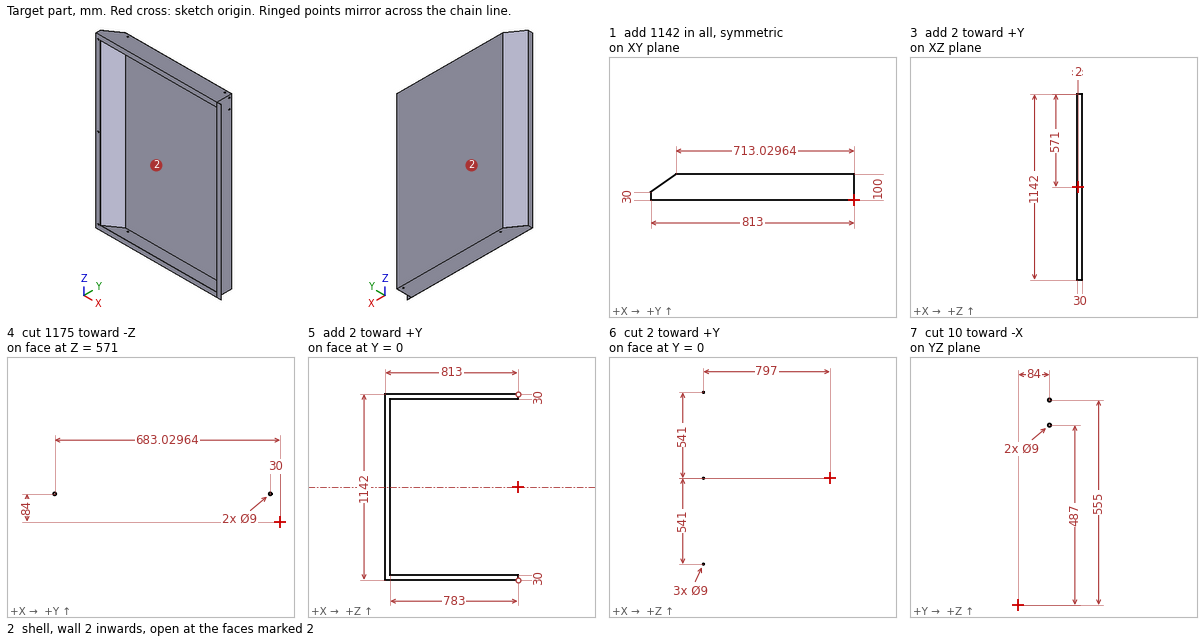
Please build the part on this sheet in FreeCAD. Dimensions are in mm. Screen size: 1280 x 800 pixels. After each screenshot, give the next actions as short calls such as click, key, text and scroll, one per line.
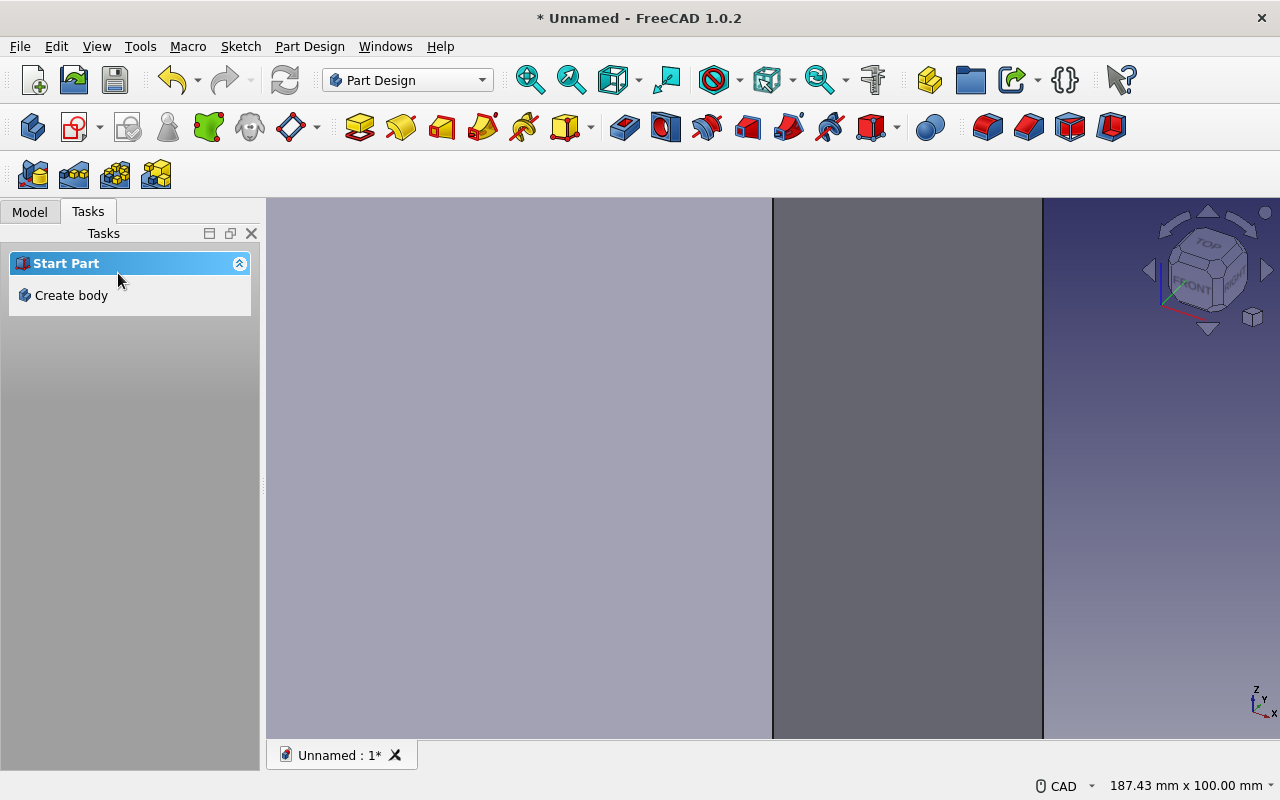
click(531, 80)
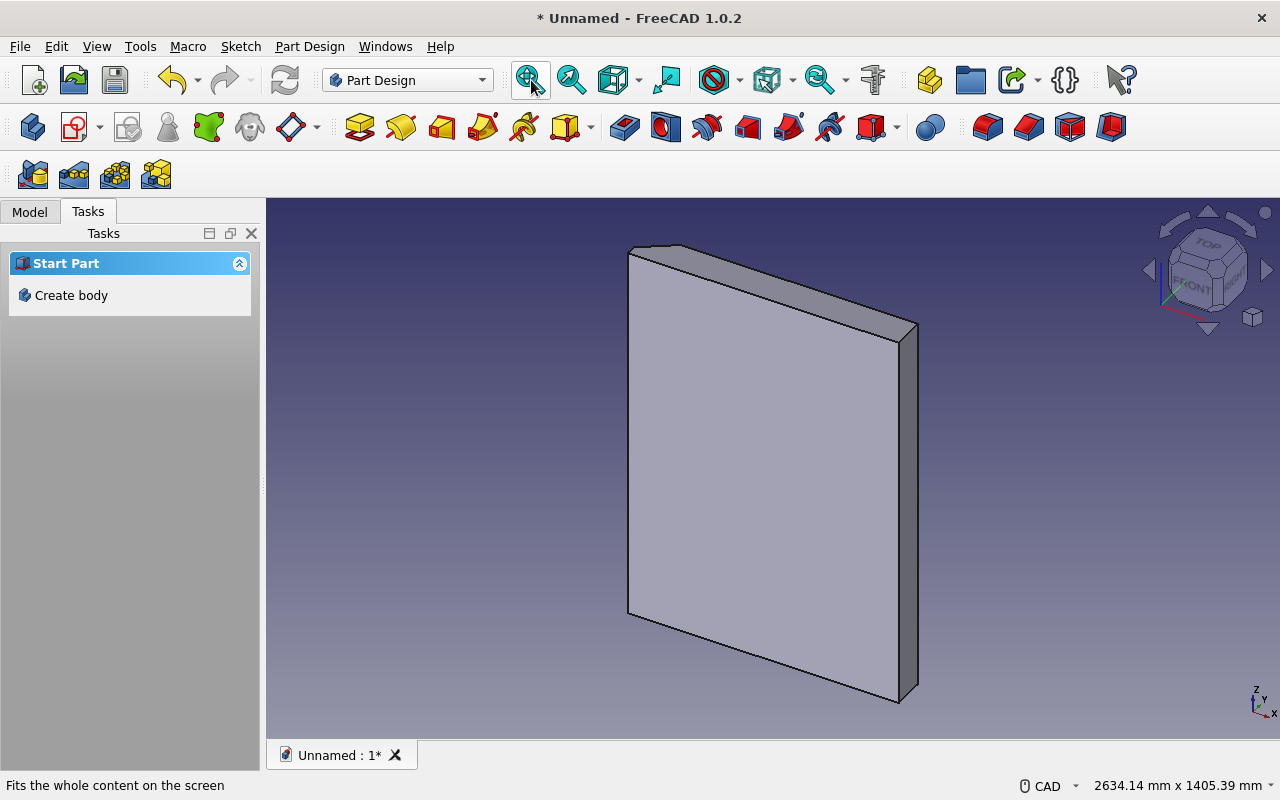
click(763, 426)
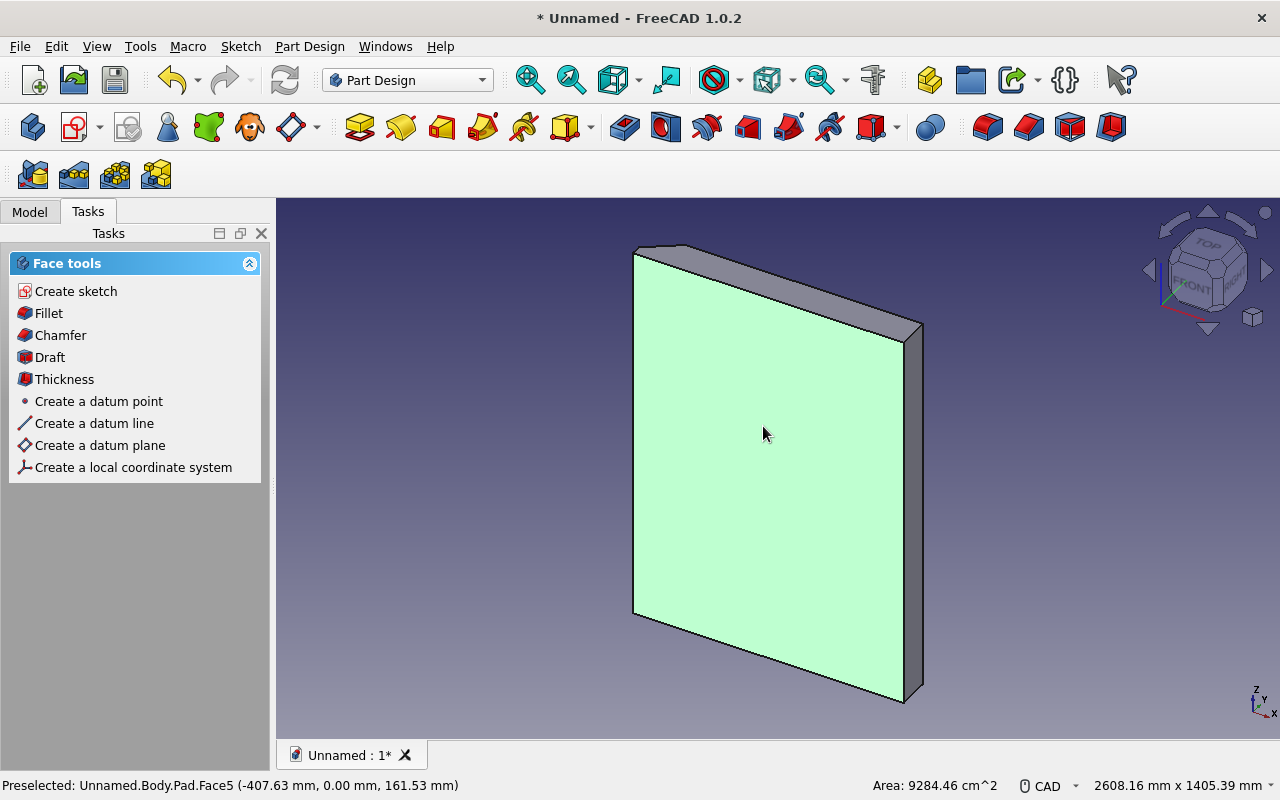
click(1111, 128)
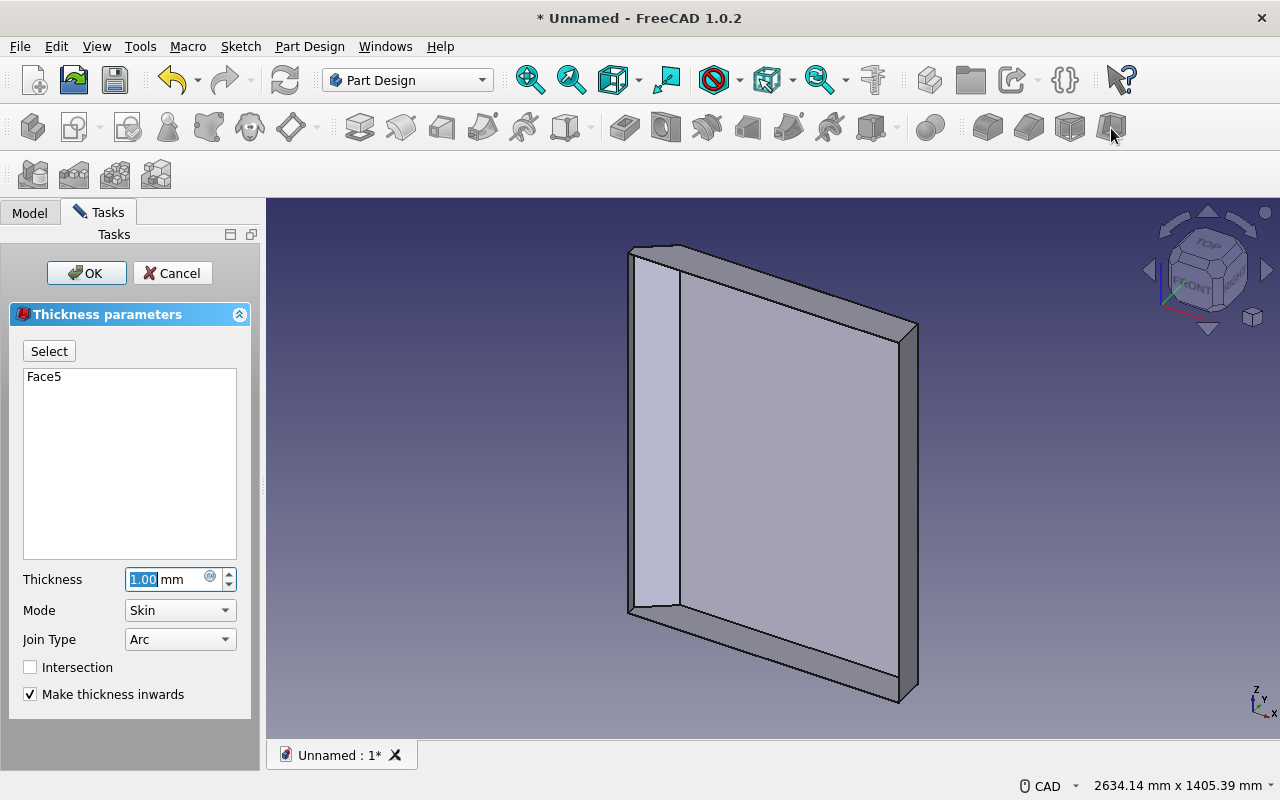
text(2)
key(Tab)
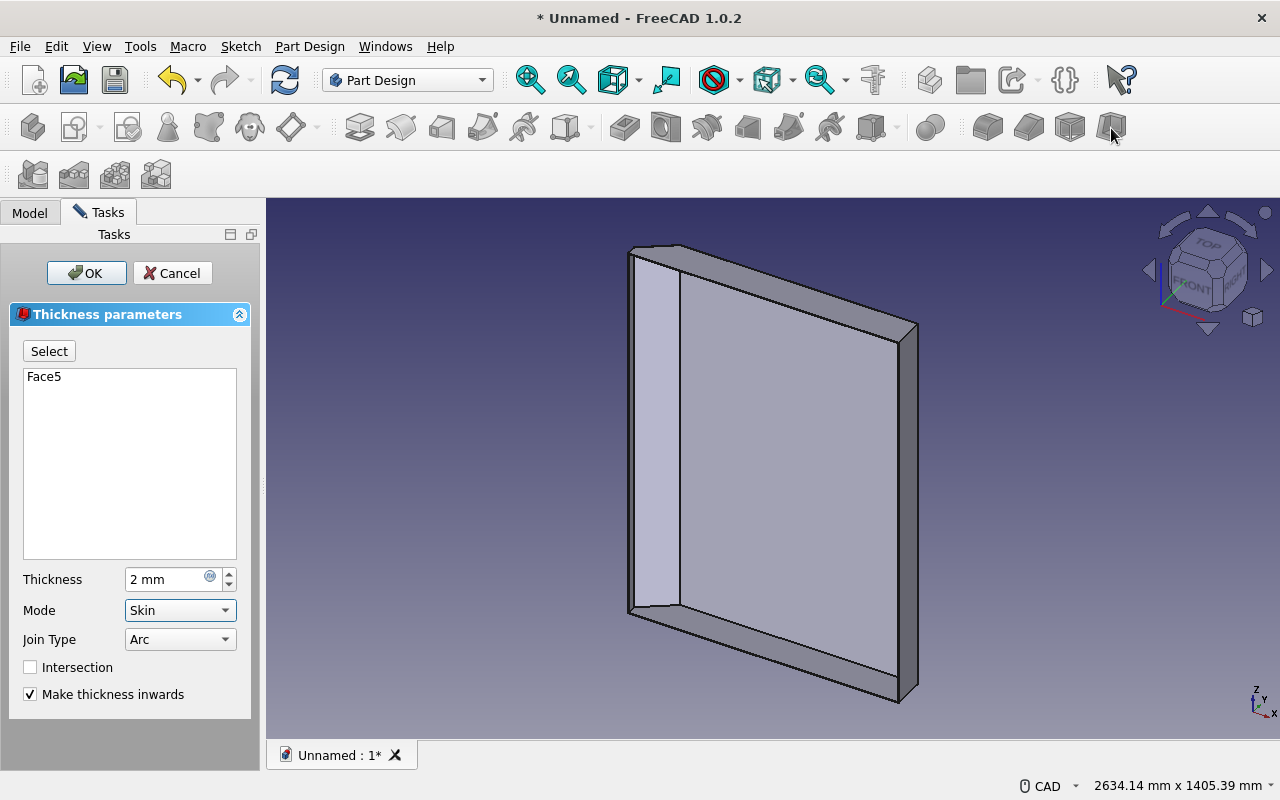
click(181, 640)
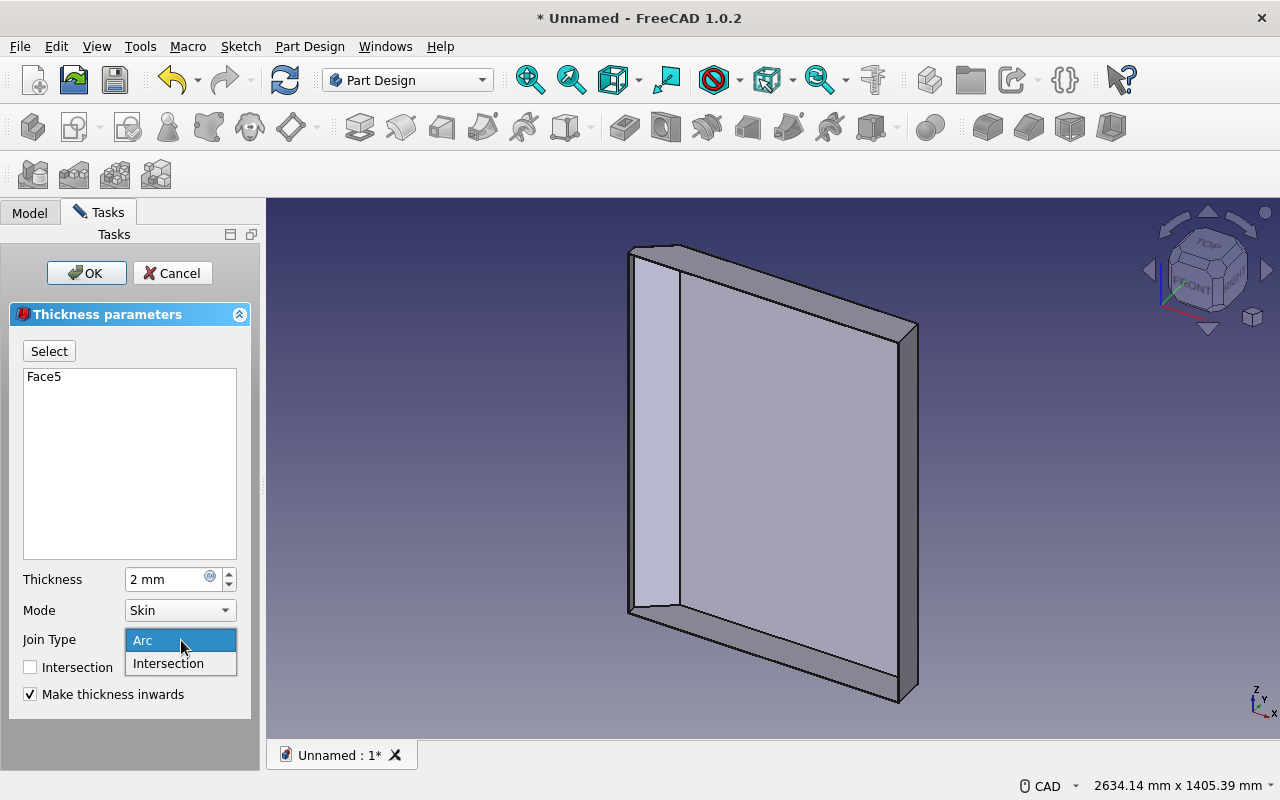
click(179, 664)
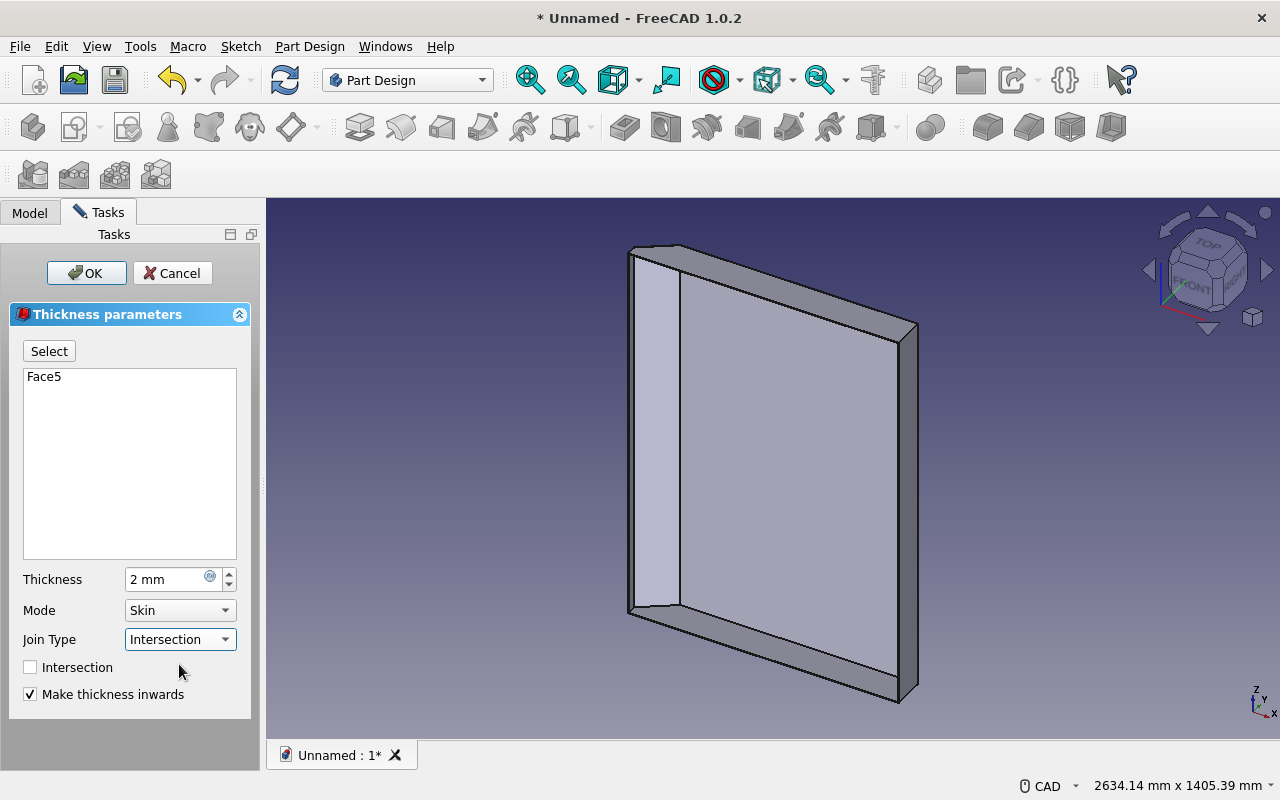
click(87, 273)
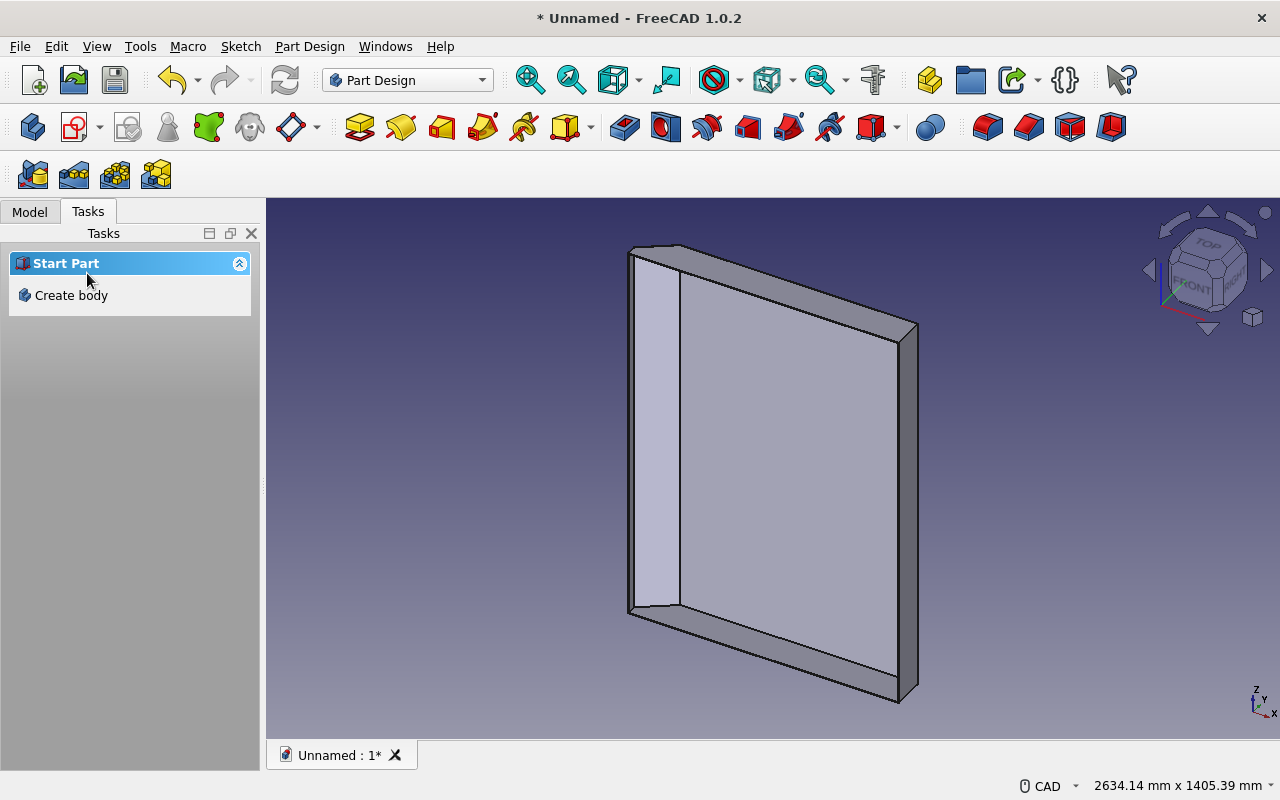
click(74, 128)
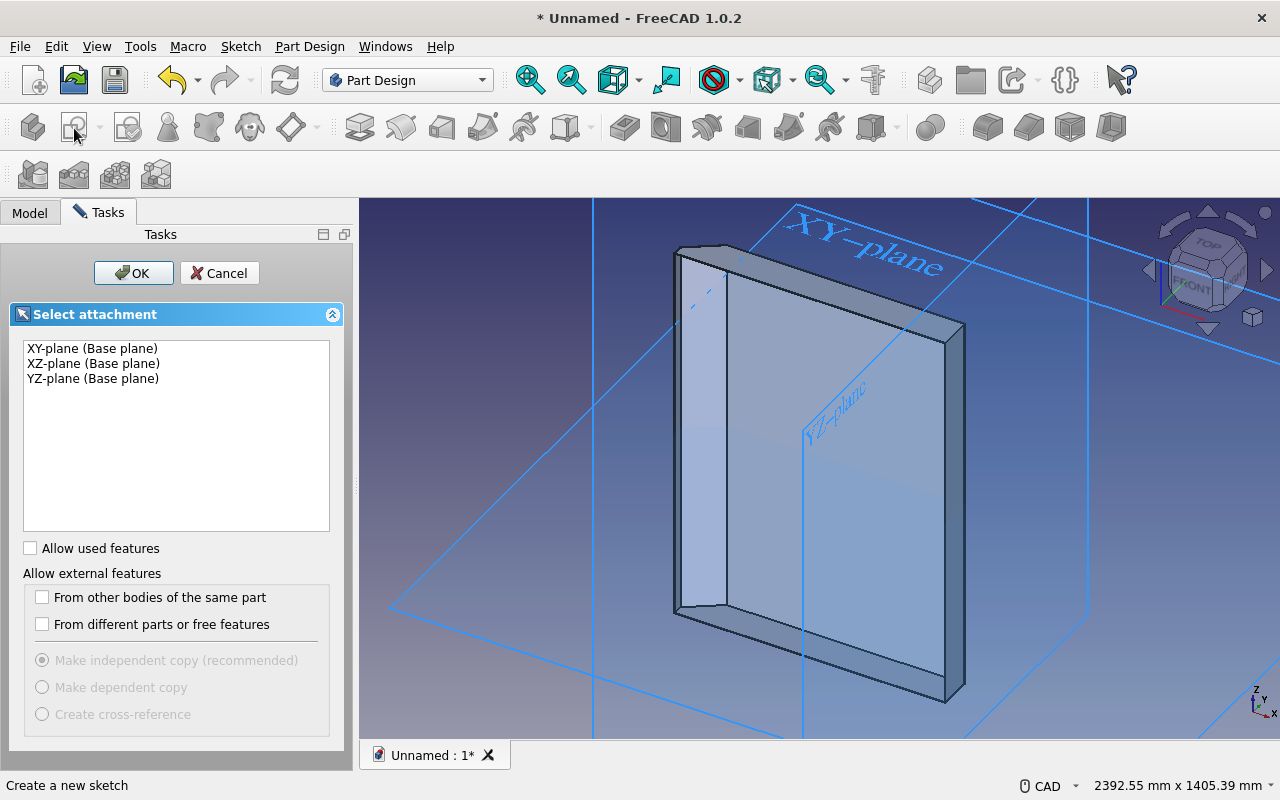
click(84, 364)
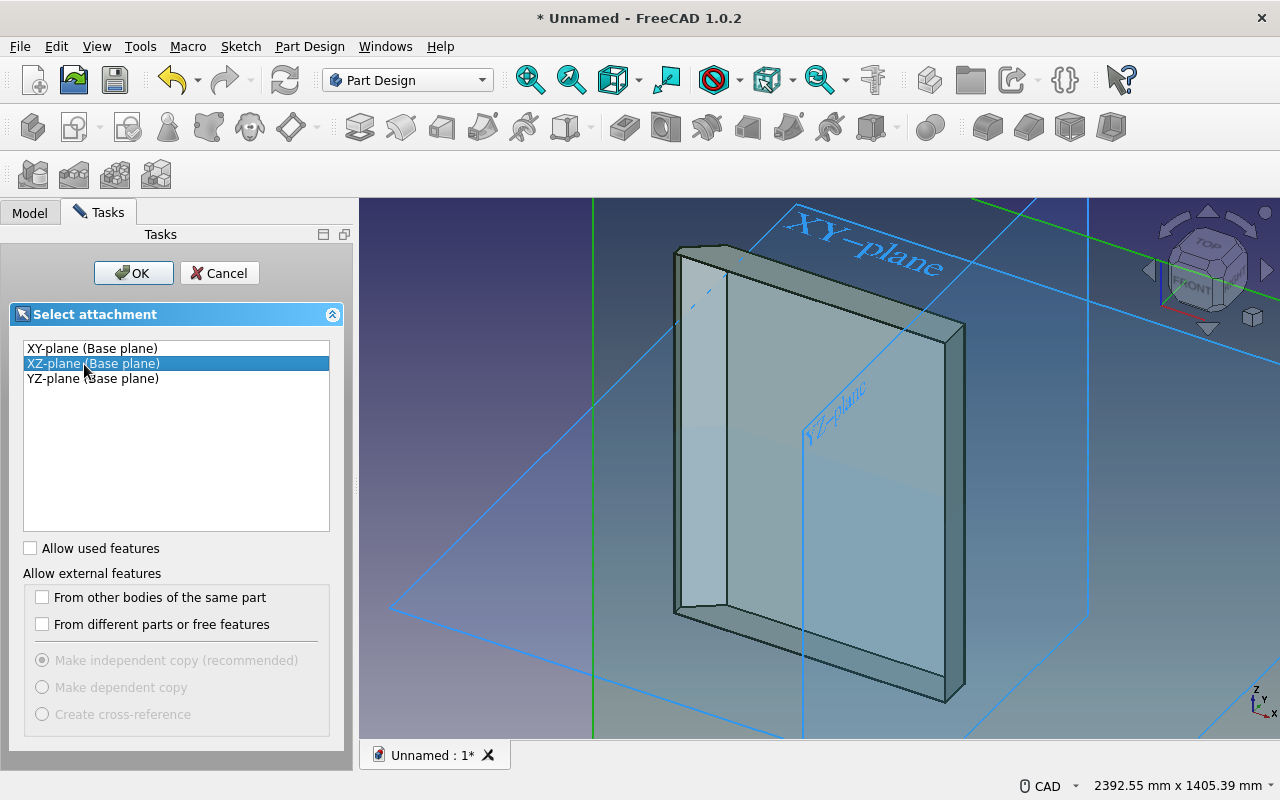
click(134, 273)